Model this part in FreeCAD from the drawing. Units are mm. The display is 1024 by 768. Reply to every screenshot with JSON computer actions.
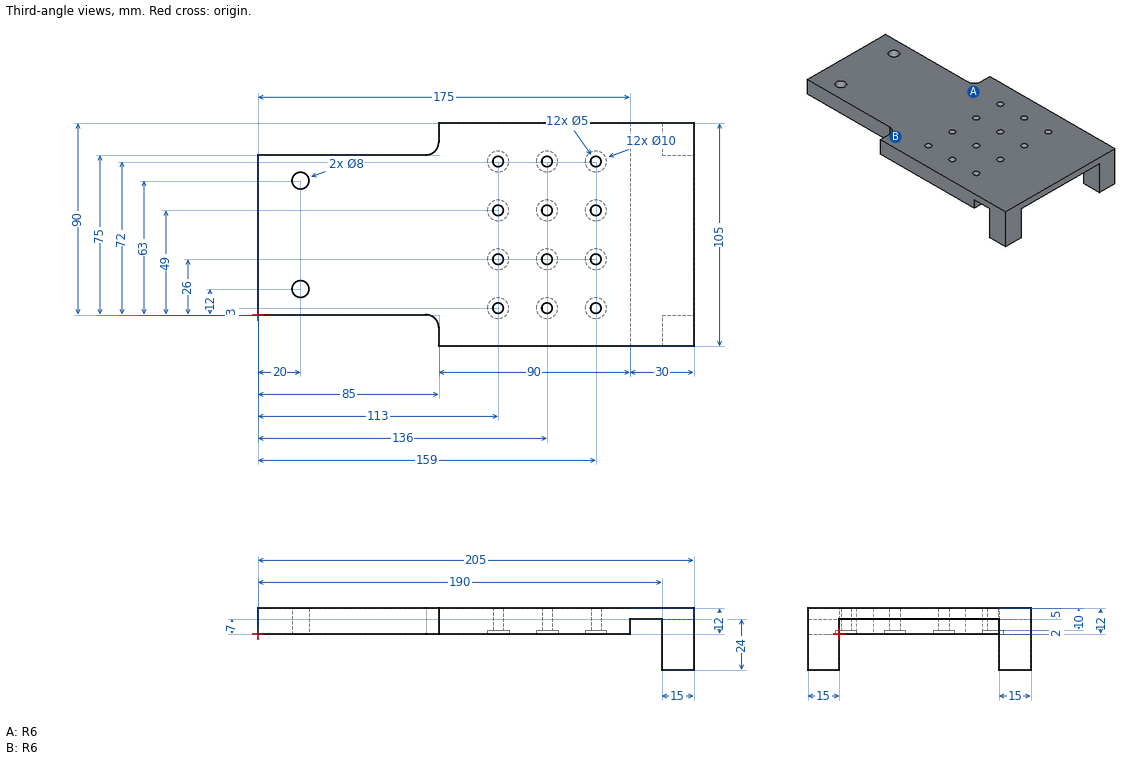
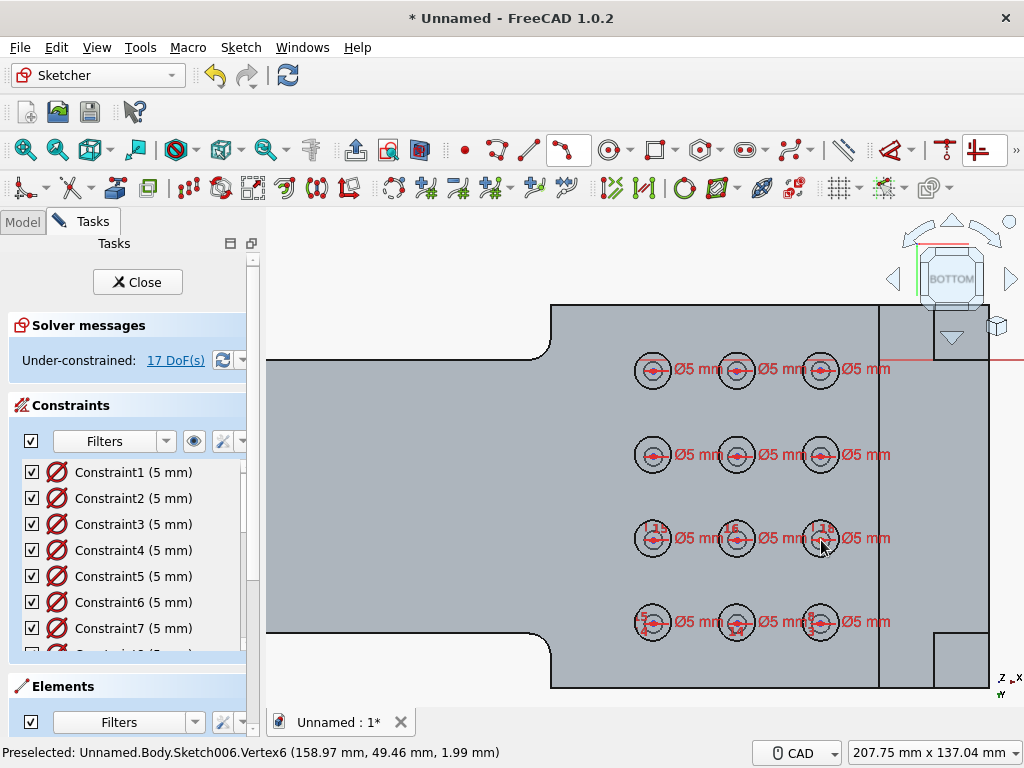
{"action": "left_click", "coordinate": [821, 457]}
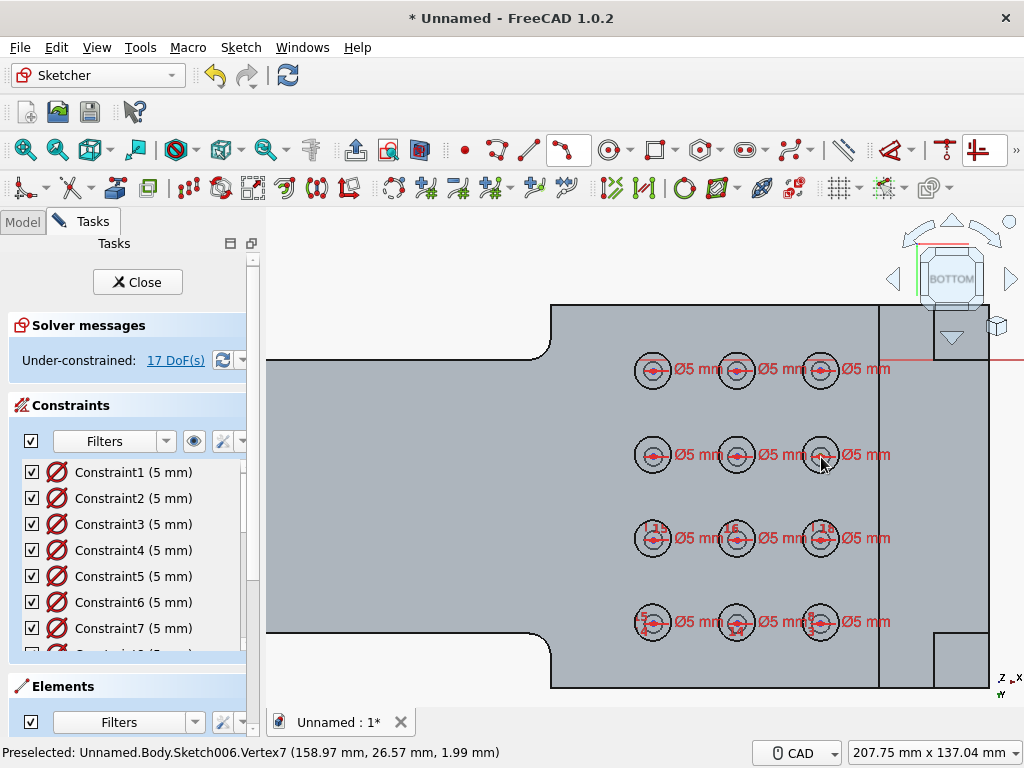
{"action": "key", "text": "v"}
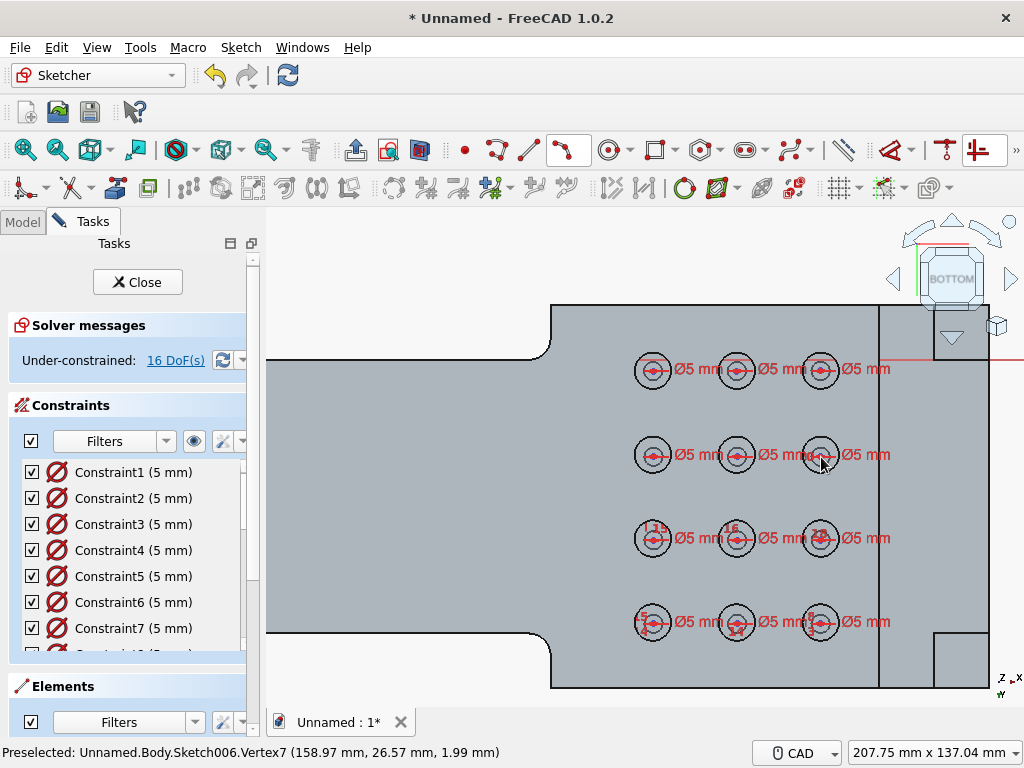
{"action": "left_click", "coordinate": [737, 540]}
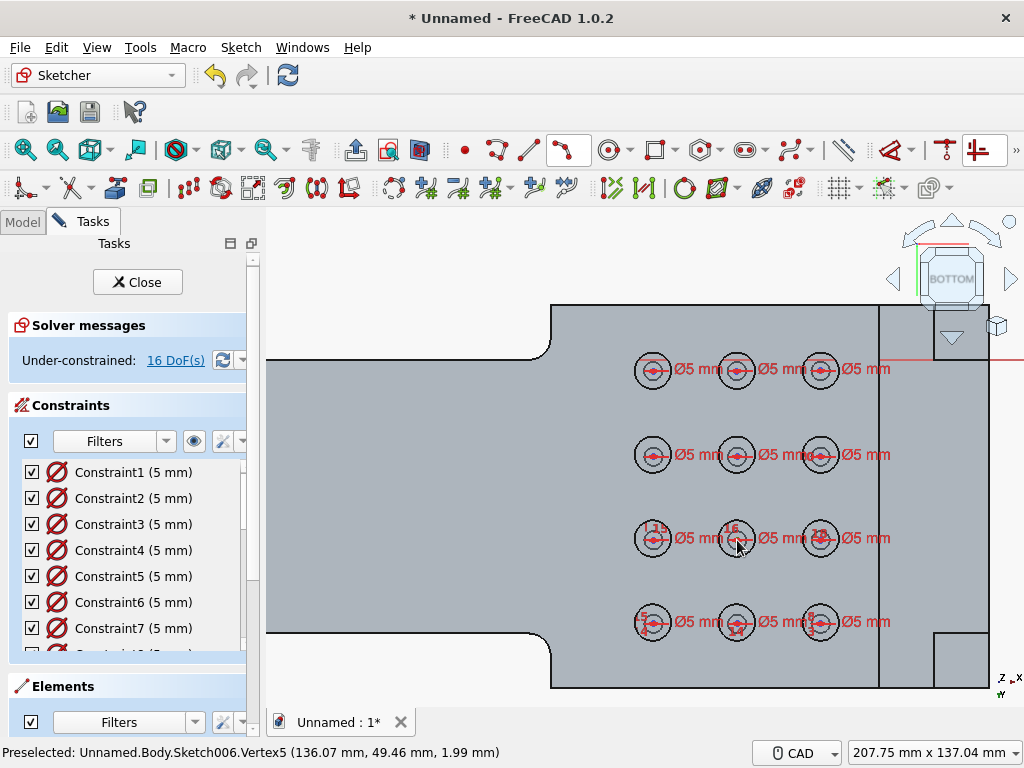
{"action": "left_click", "coordinate": [737, 457]}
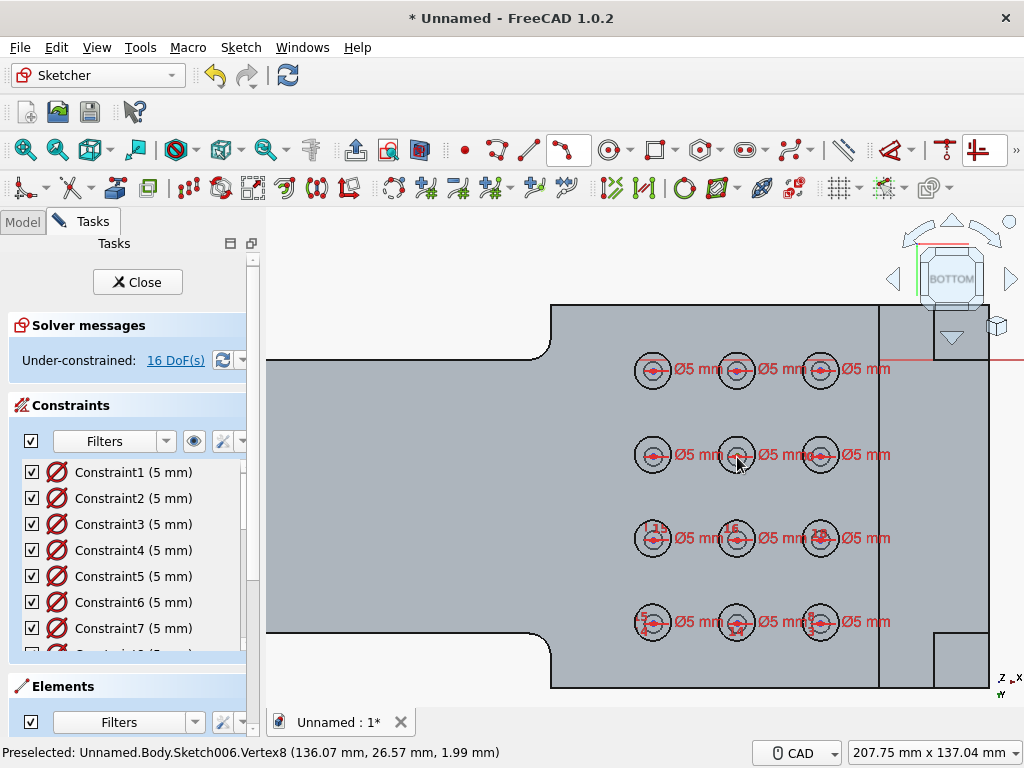
{"action": "left_click", "coordinate": [1002, 150]}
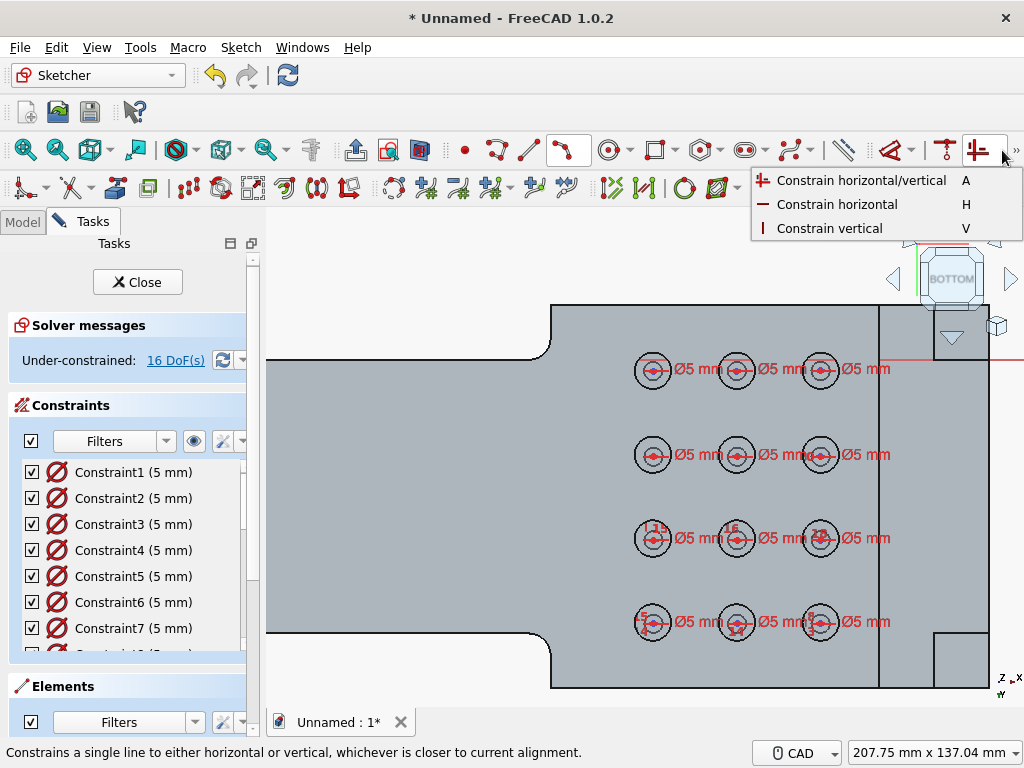
{"action": "left_click", "coordinate": [887, 228]}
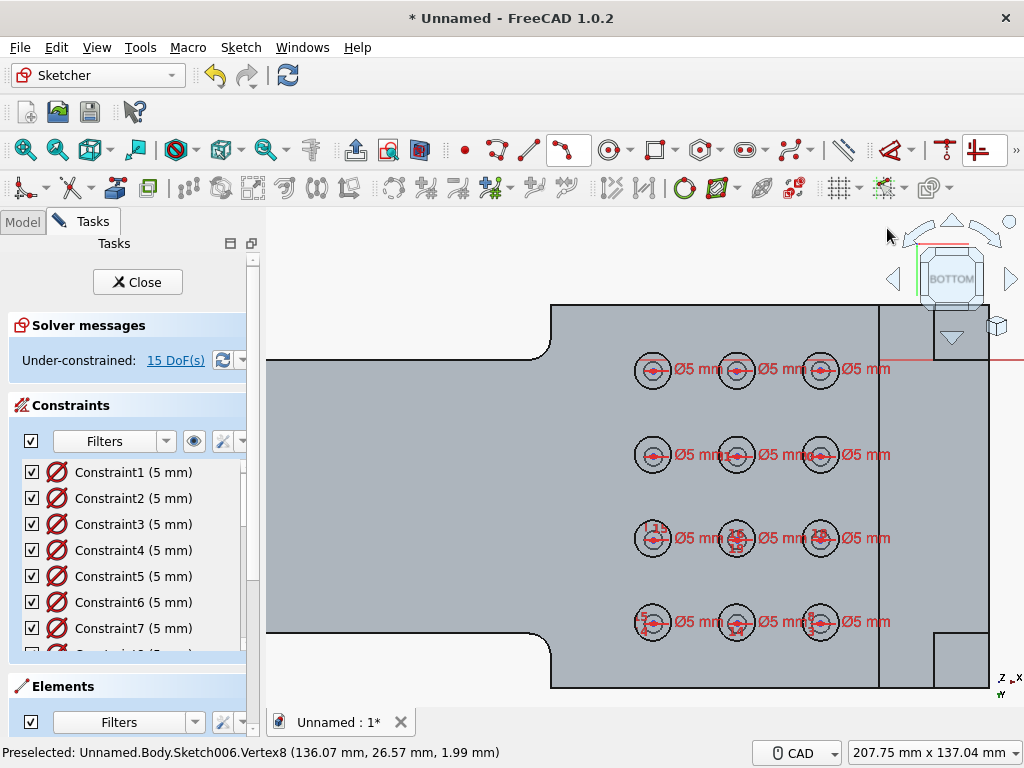
{"action": "left_click", "coordinate": [821, 457]}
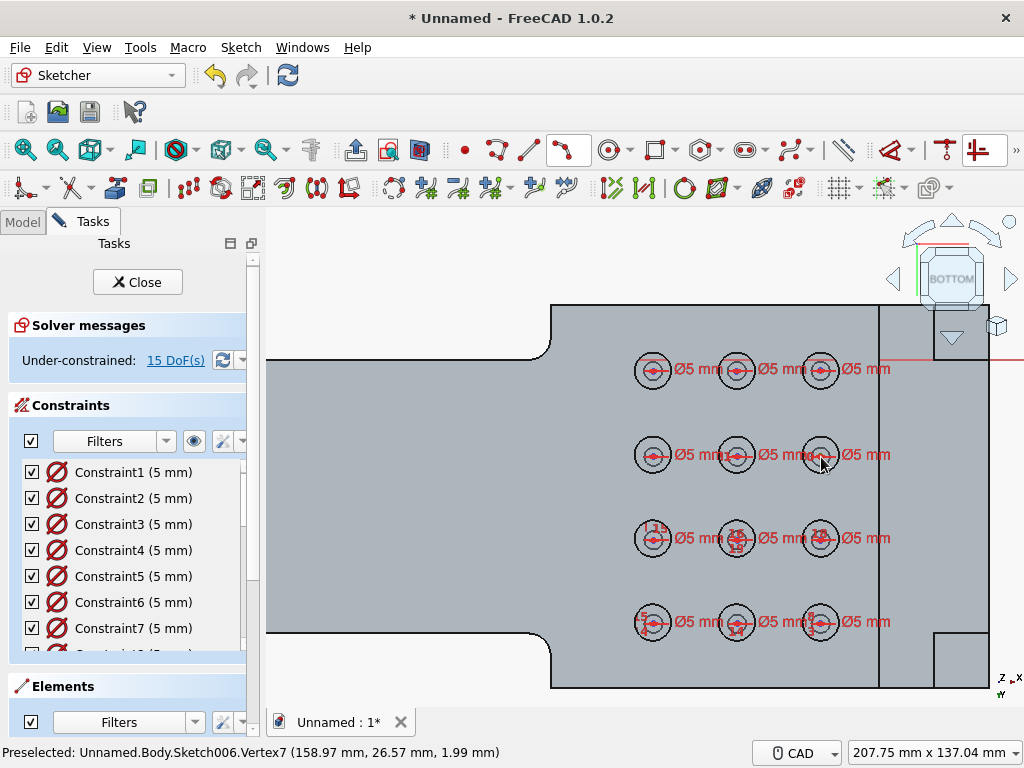
{"action": "left_click", "coordinate": [737, 457]}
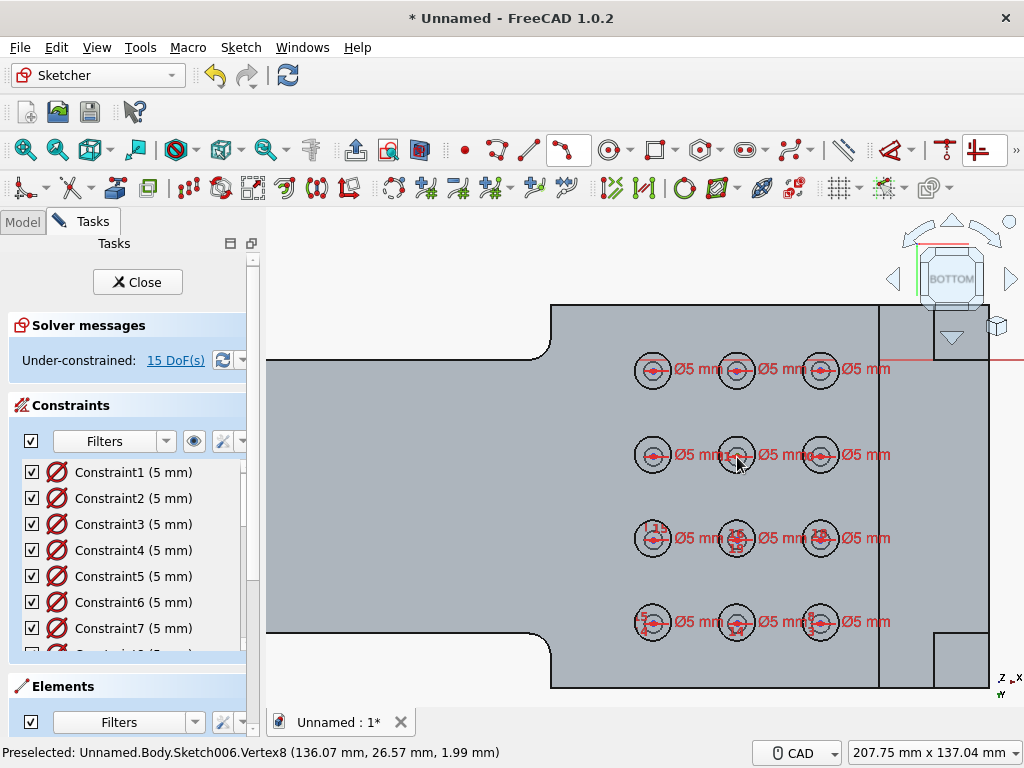
{"action": "key", "text": "h"}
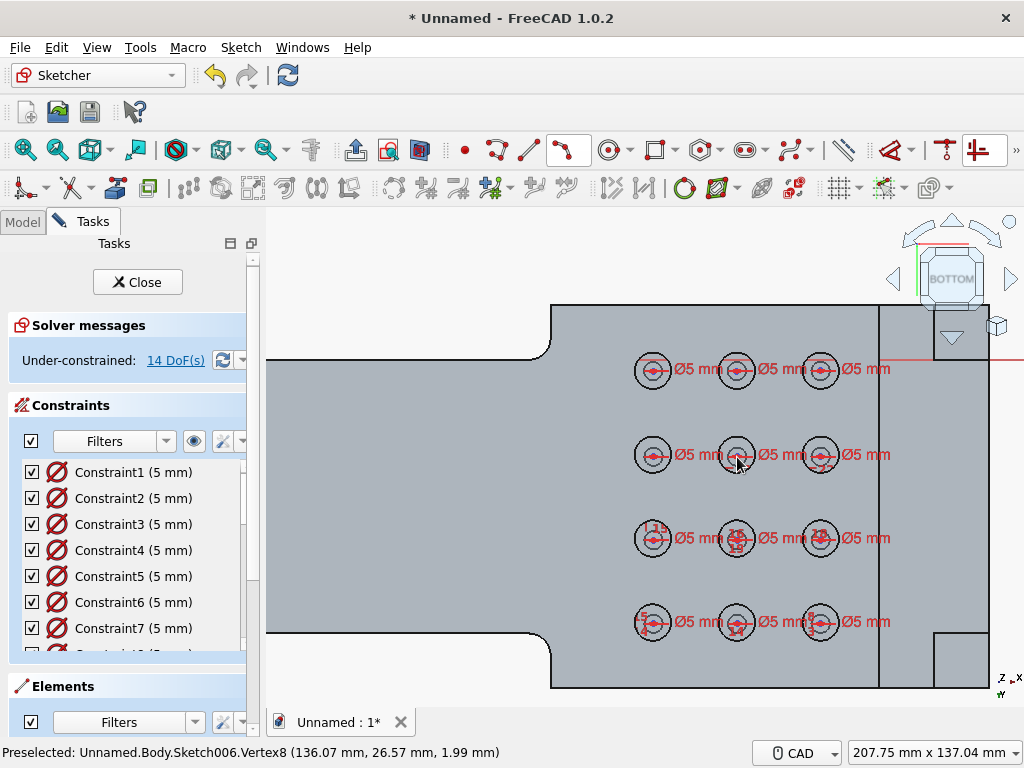
{"action": "left_click", "coordinate": [654, 540]}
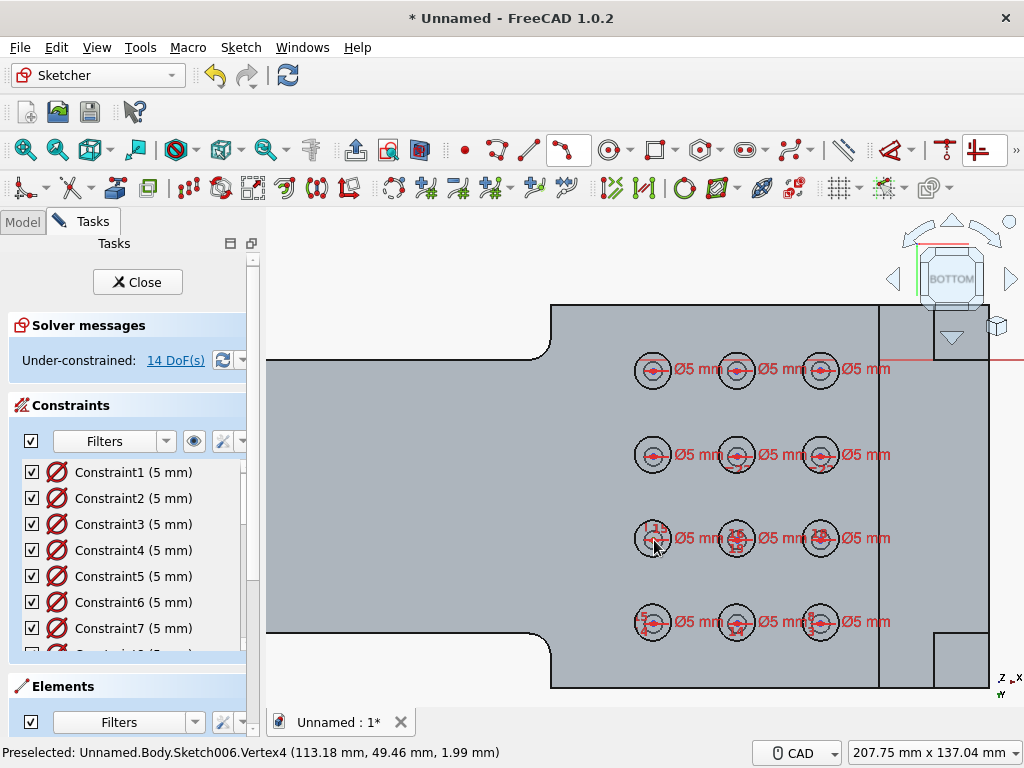
{"action": "left_click", "coordinate": [654, 457]}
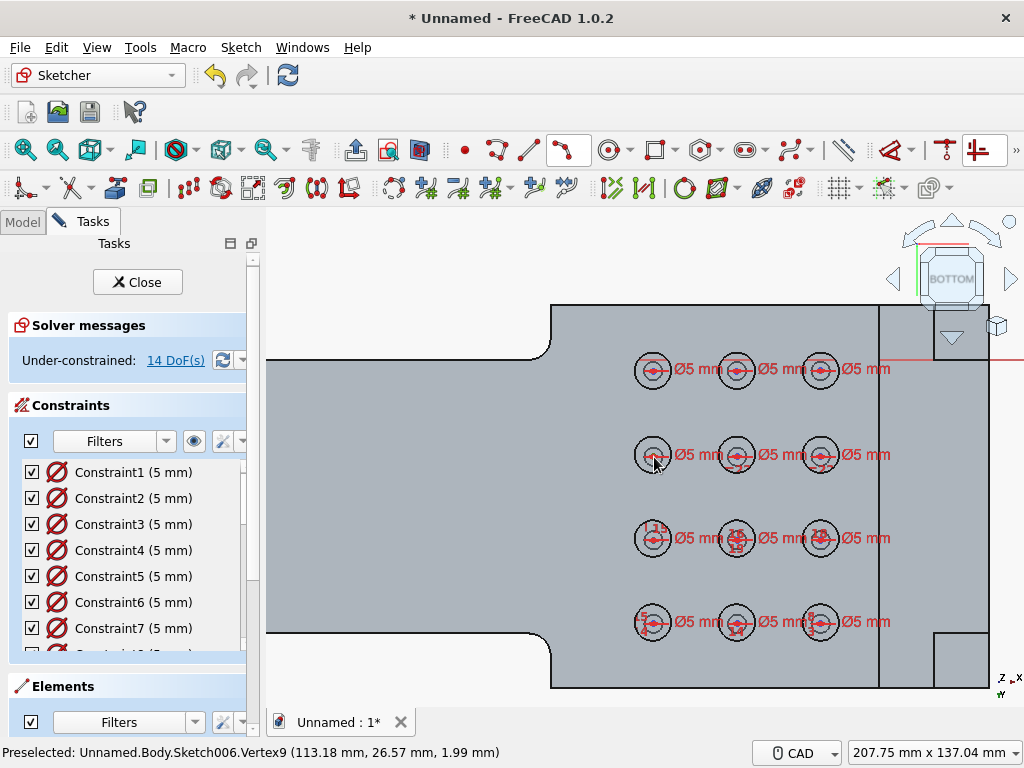
{"action": "left_click", "coordinate": [1002, 150]}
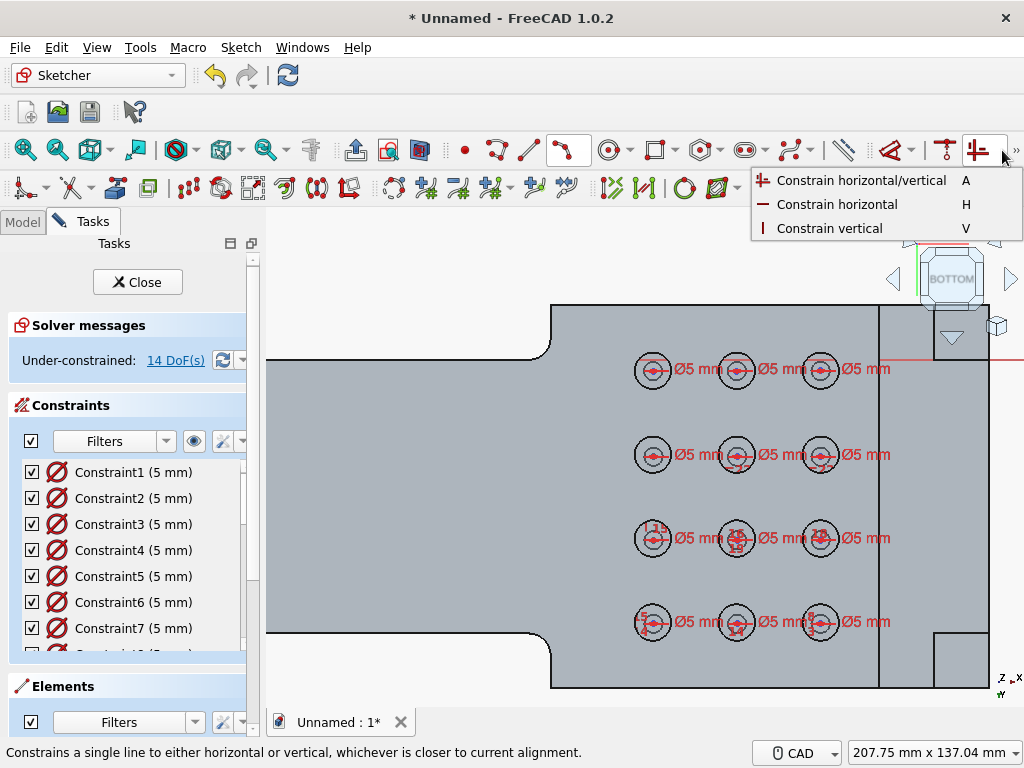
{"action": "left_click", "coordinate": [887, 228]}